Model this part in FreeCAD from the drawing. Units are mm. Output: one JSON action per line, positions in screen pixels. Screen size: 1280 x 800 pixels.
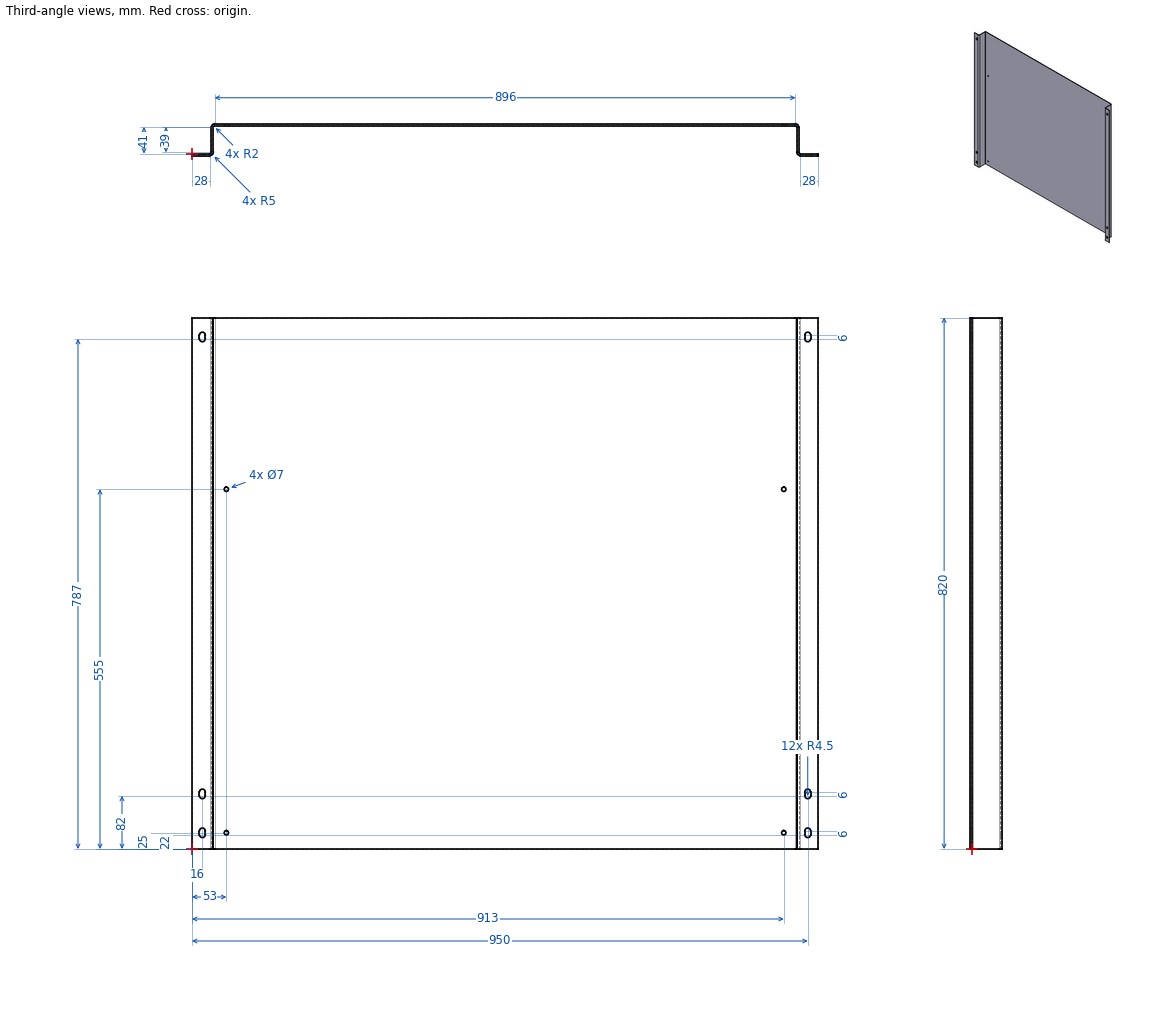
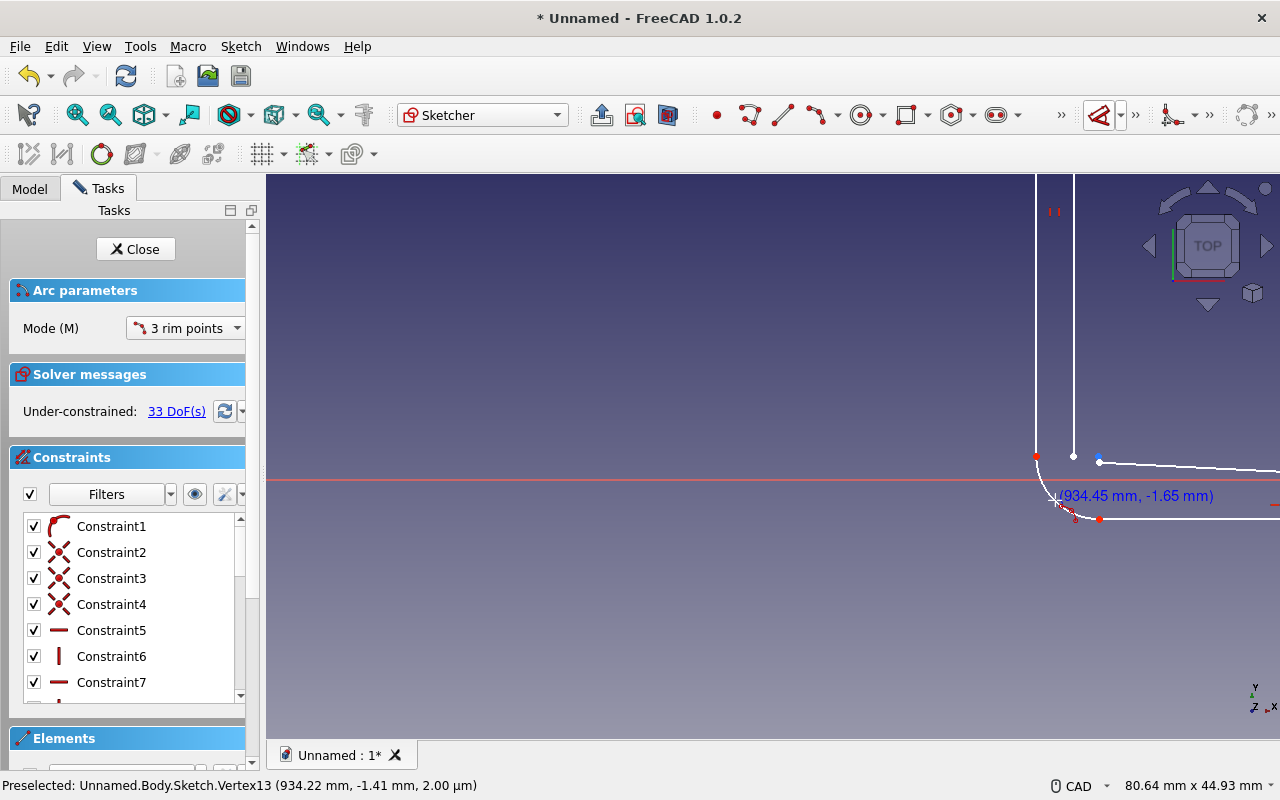
{"action": "left_click", "coordinate": [1099, 463]}
{"action": "left_click", "coordinate": [1074, 456]}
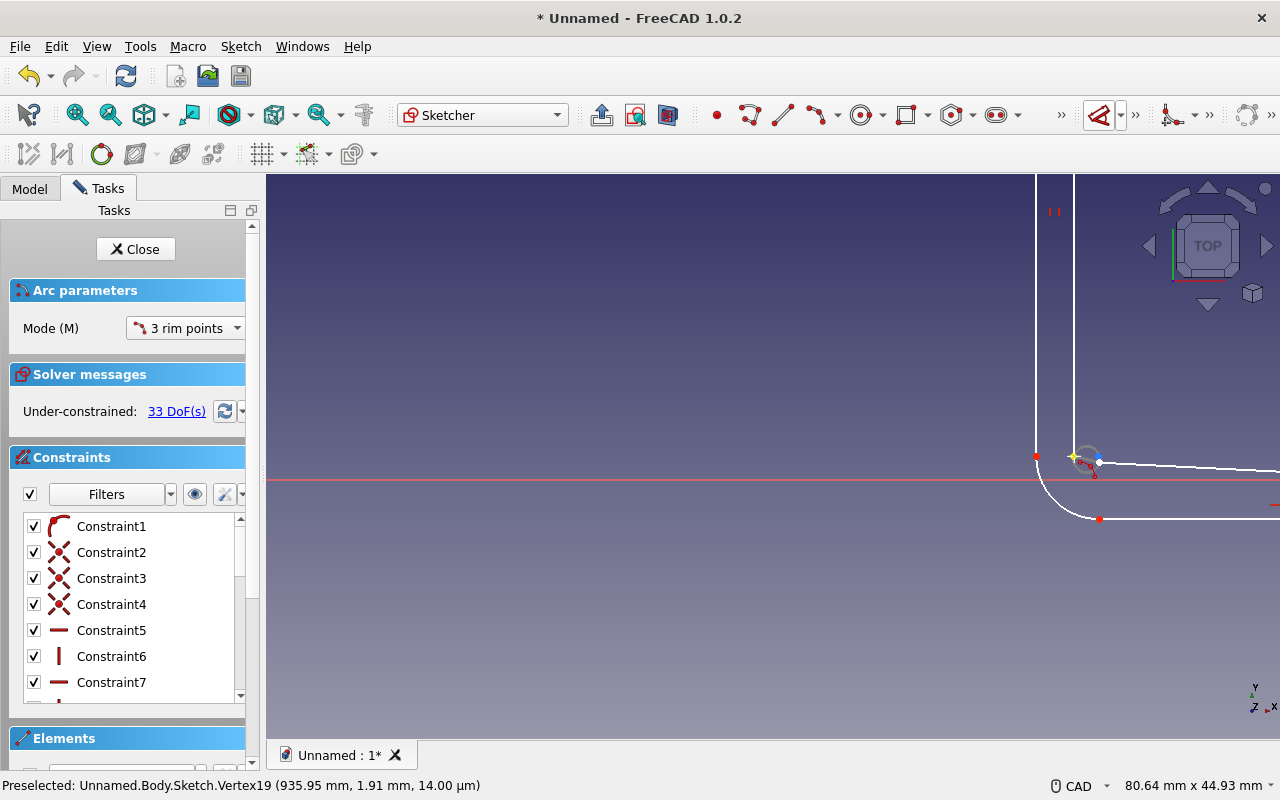
{"action": "scroll", "coordinate": [1082, 473], "scroll_direction": "up", "scroll_amount": 4}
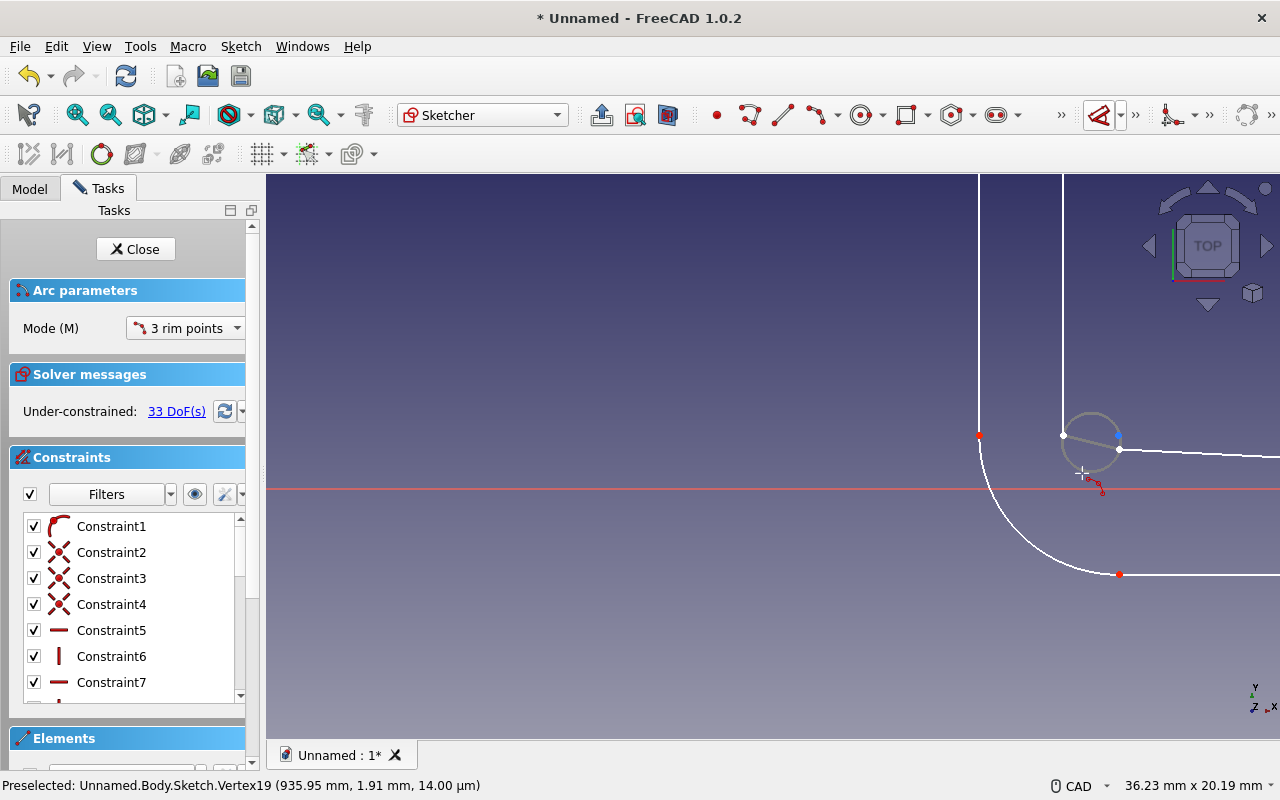
{"action": "left_click", "coordinate": [1081, 472]}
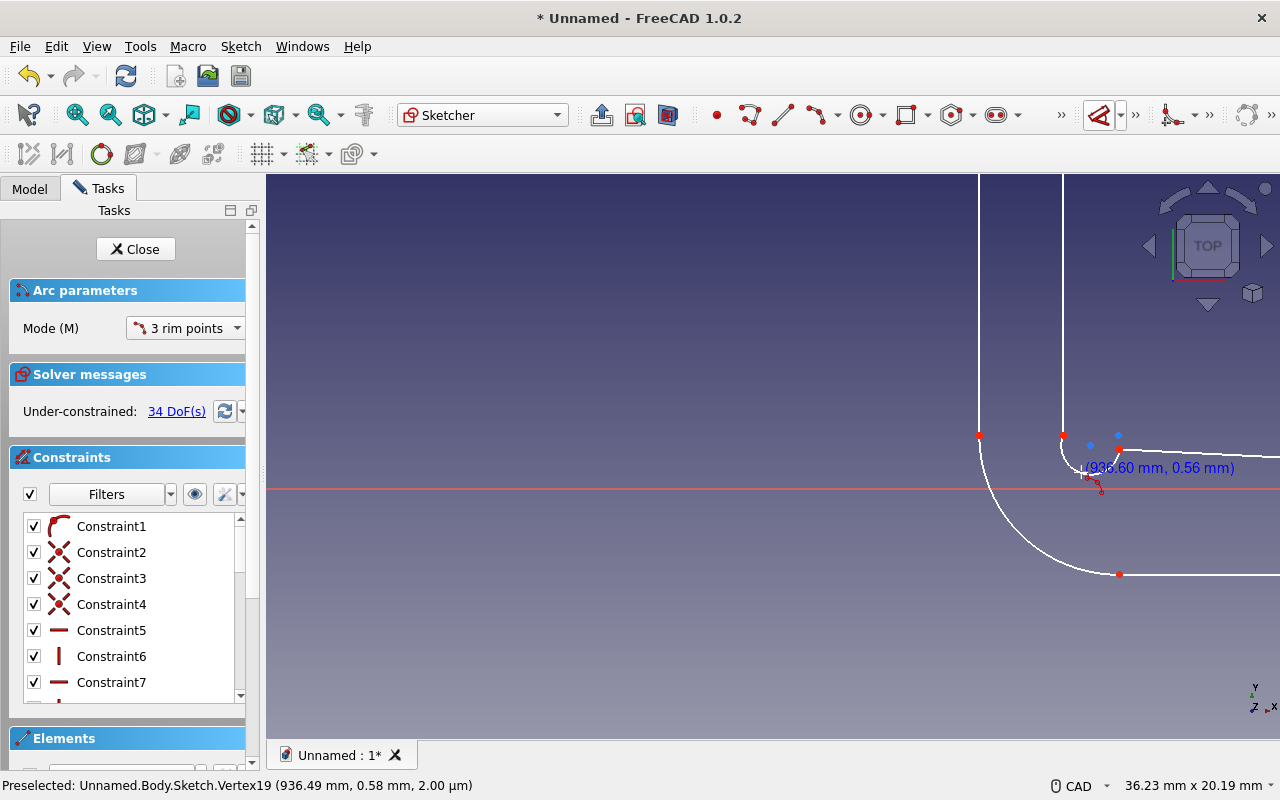
{"action": "scroll", "coordinate": [1051, 472], "scroll_direction": "down", "scroll_amount": 18}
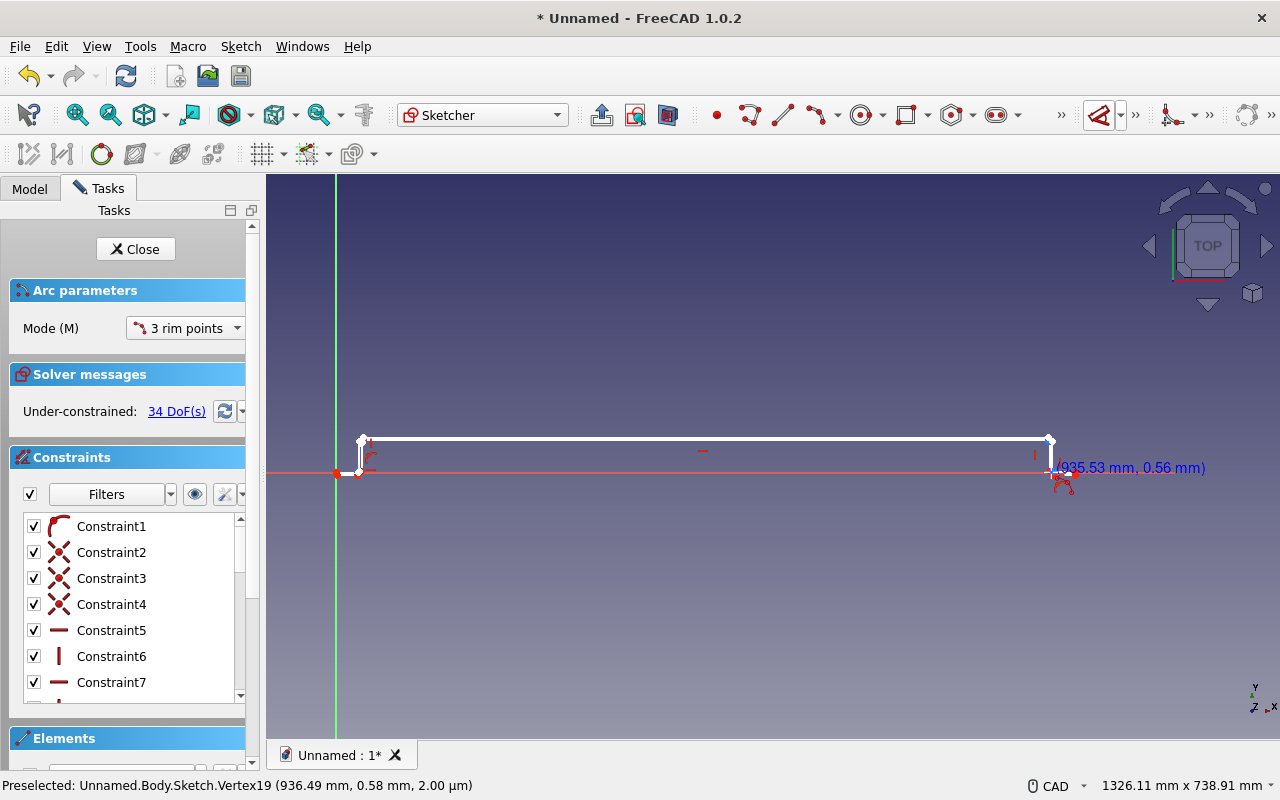
{"action": "scroll", "coordinate": [1052, 442], "scroll_direction": "up", "scroll_amount": 10}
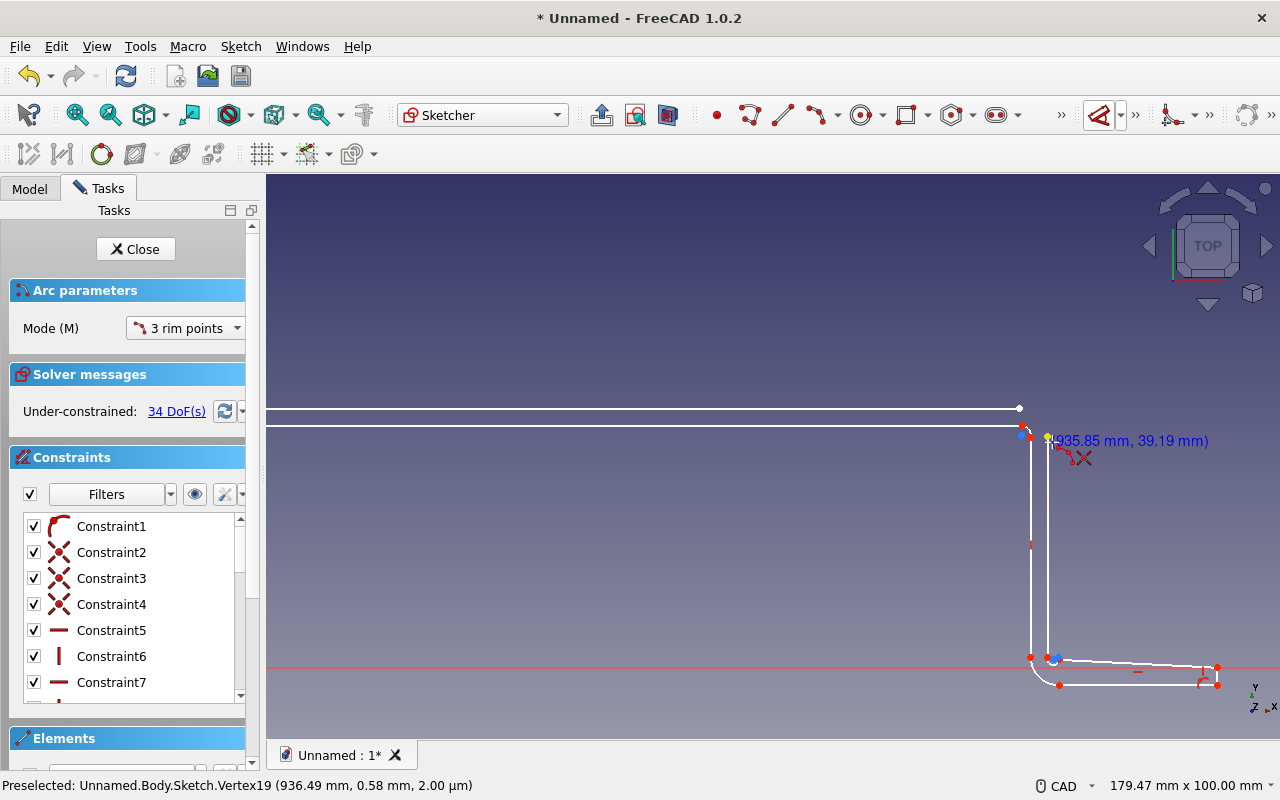
{"action": "left_click", "coordinate": [1048, 437]}
{"action": "left_click", "coordinate": [1020, 409]}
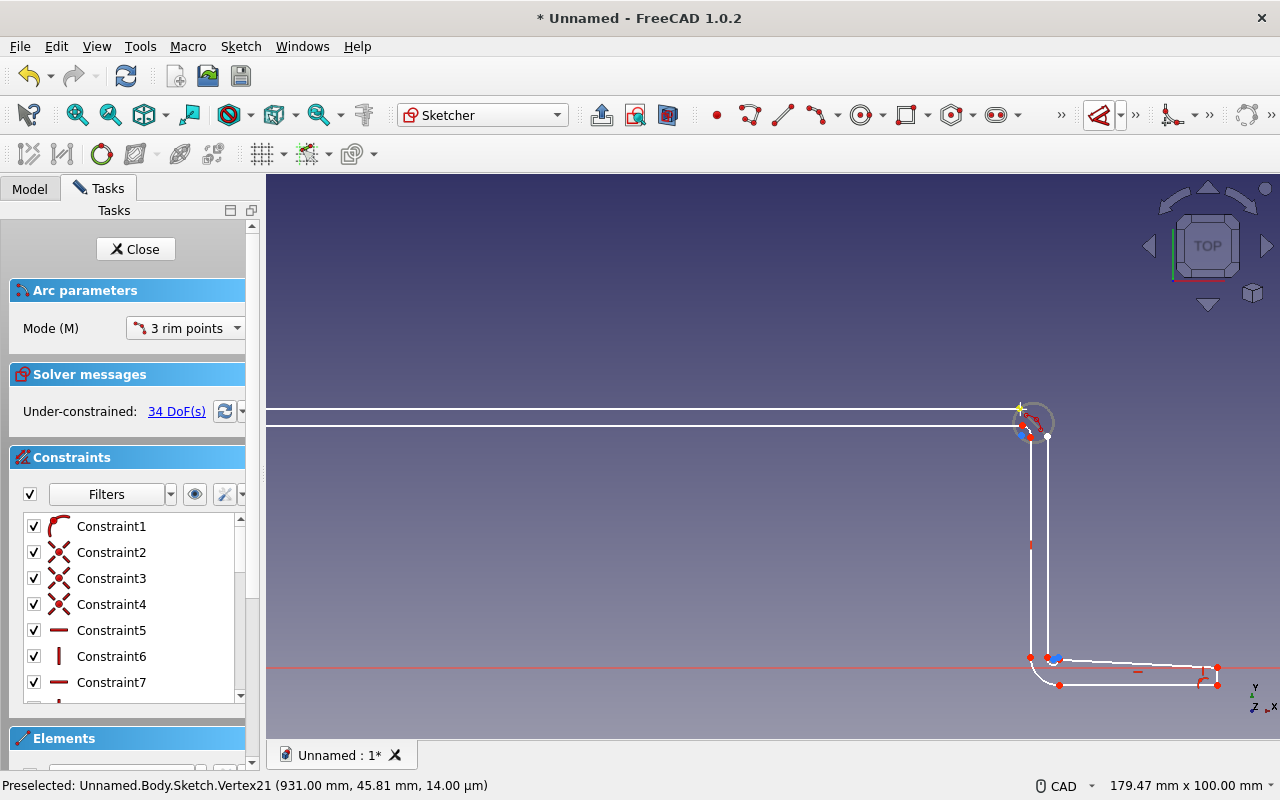
{"action": "scroll", "coordinate": [1040, 416], "scroll_direction": "up", "scroll_amount": 4}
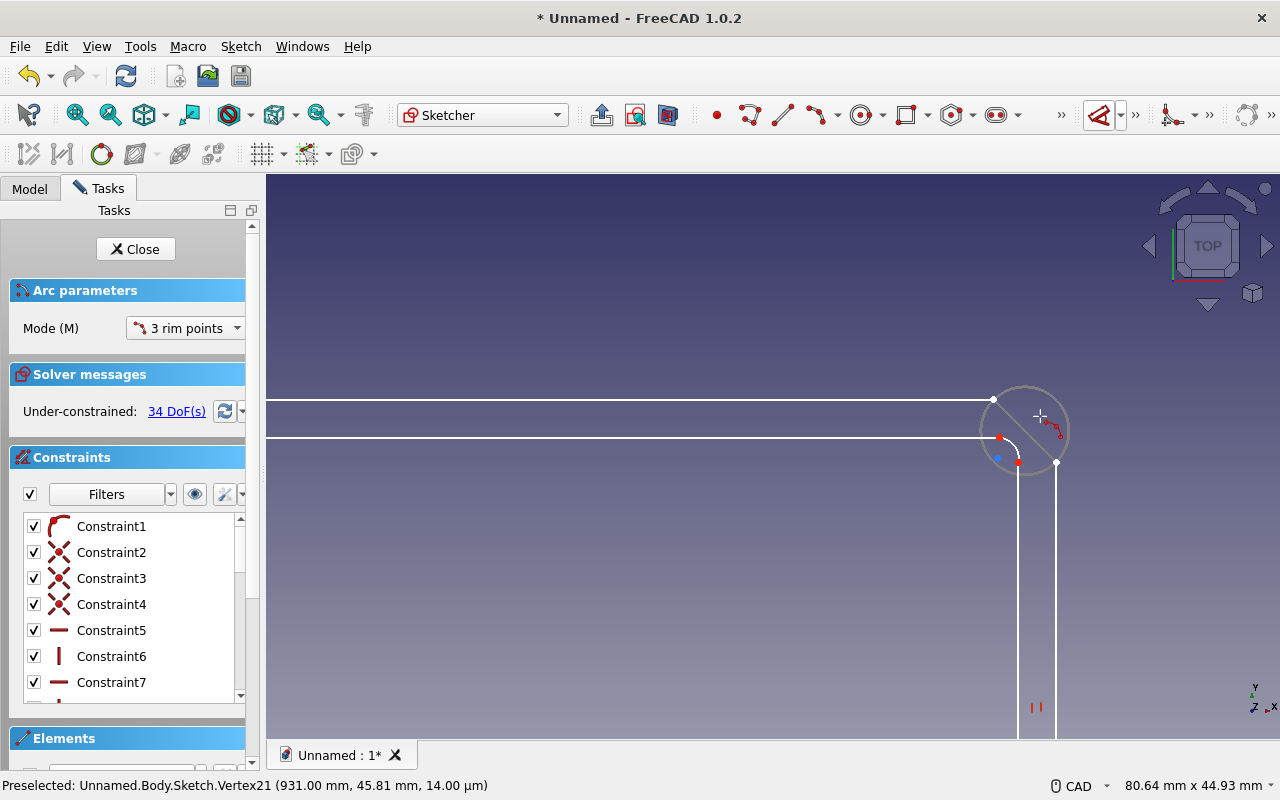
{"action": "left_click", "coordinate": [1038, 416]}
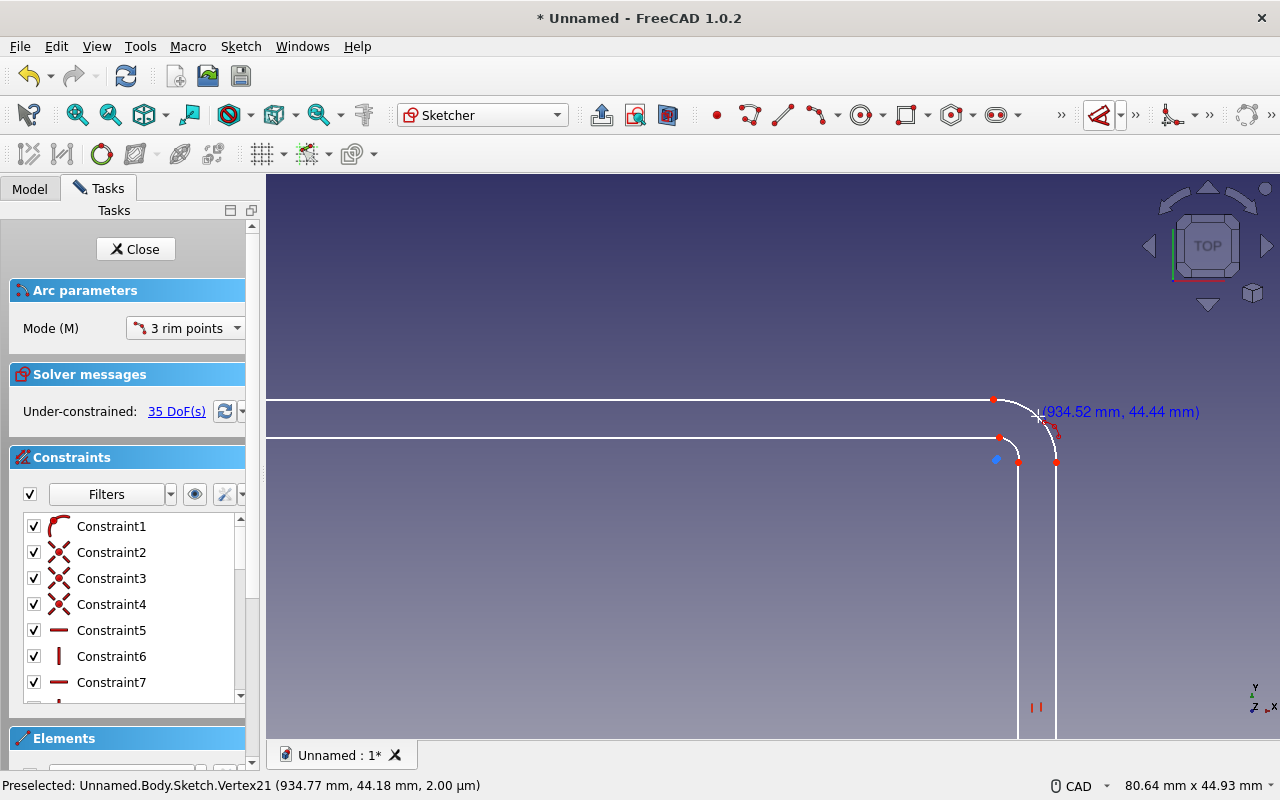
{"action": "scroll", "coordinate": [985, 443], "scroll_direction": "down", "scroll_amount": 15}